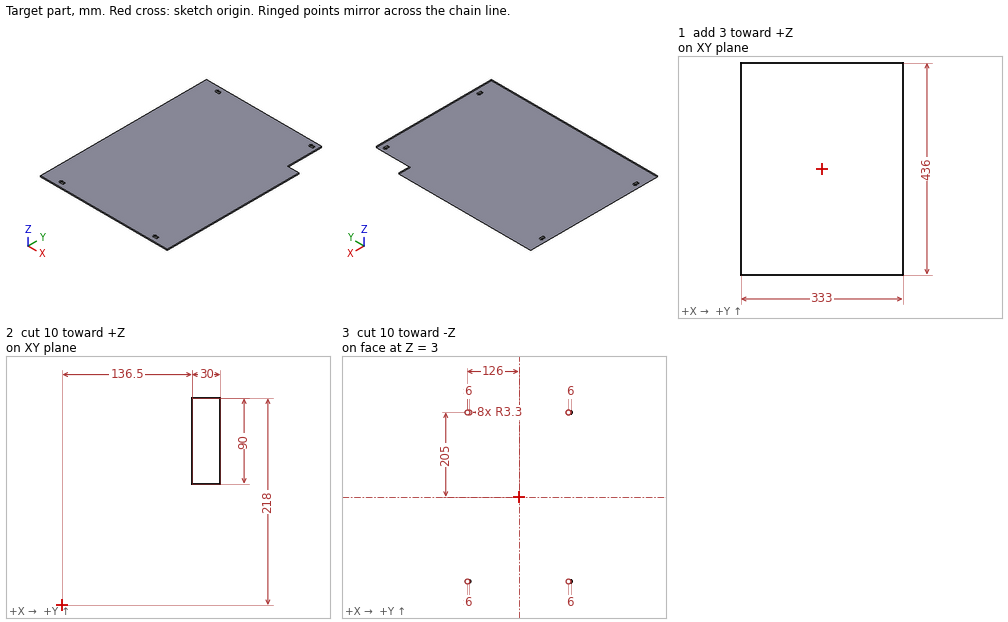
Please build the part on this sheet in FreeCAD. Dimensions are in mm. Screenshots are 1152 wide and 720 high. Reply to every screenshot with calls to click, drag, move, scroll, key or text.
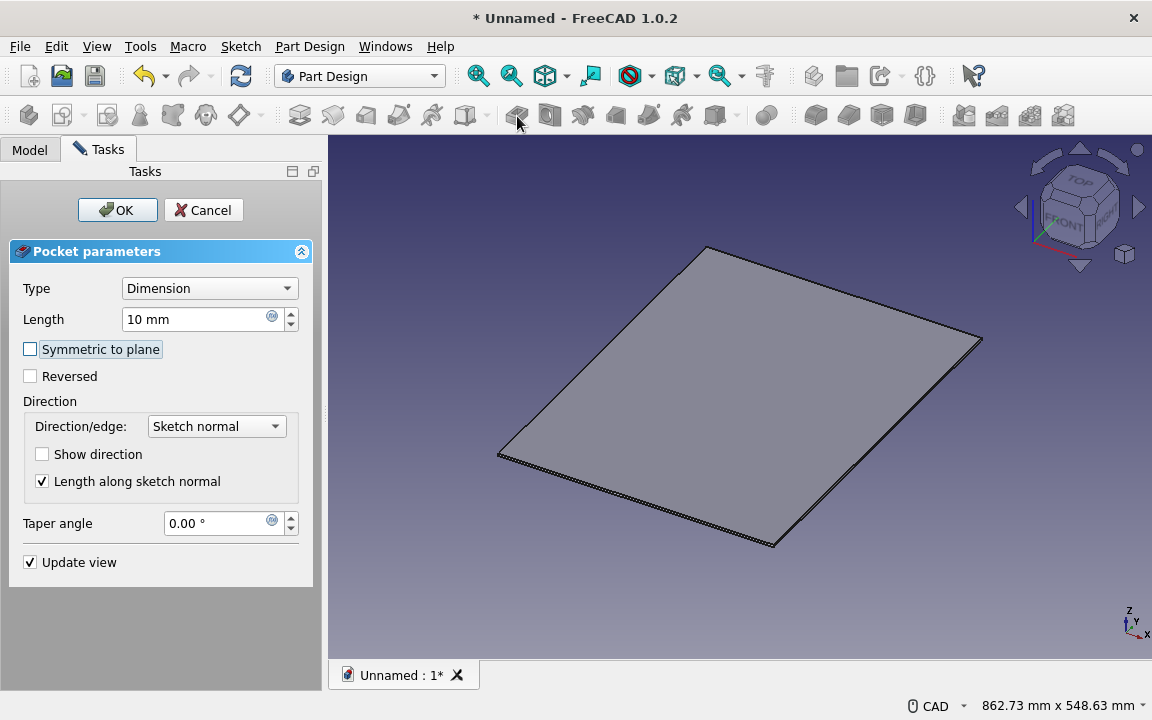
click(31, 376)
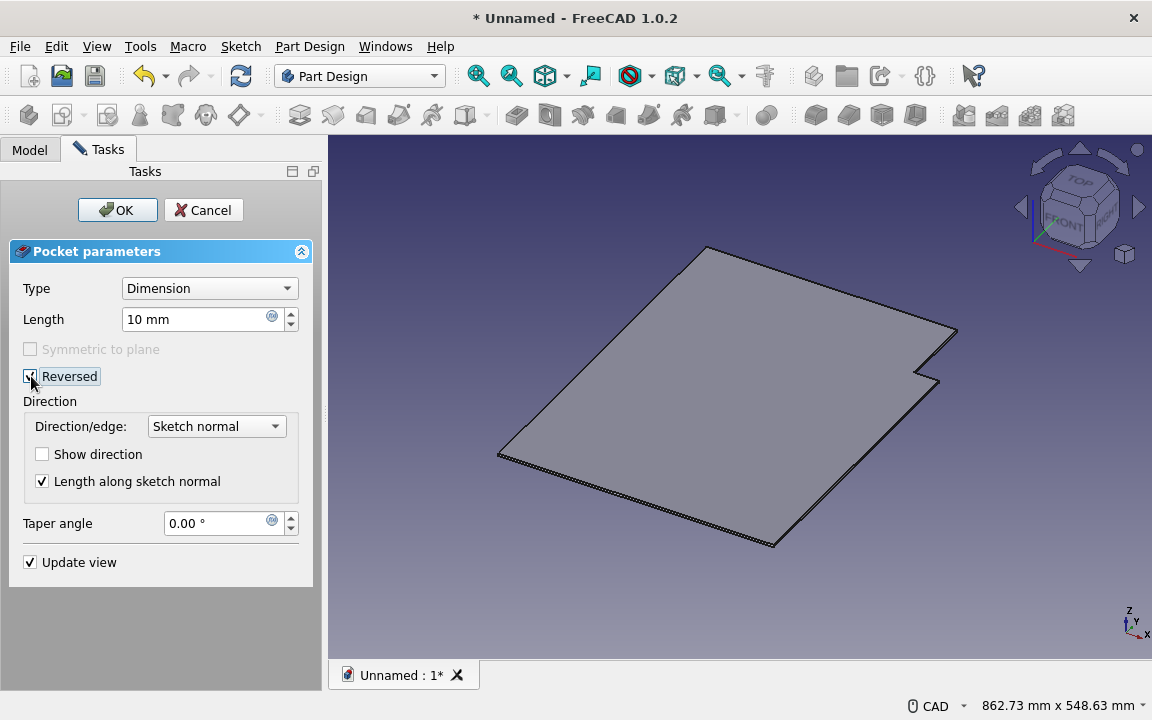
click(118, 210)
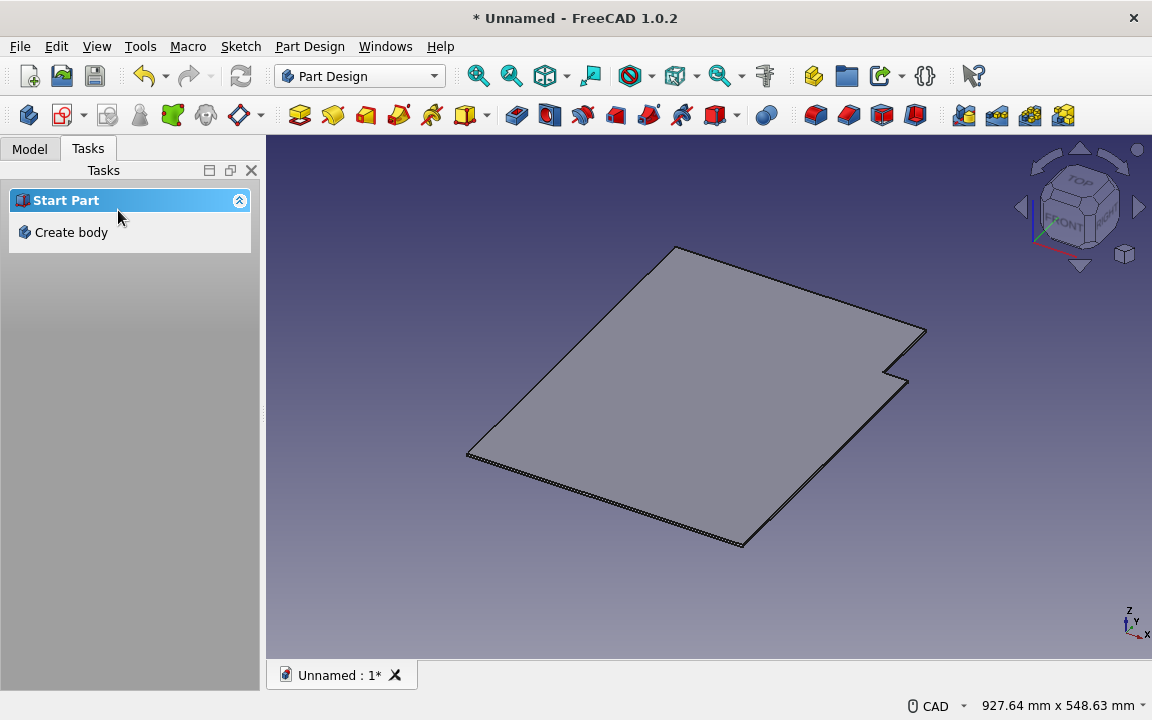
click(709, 395)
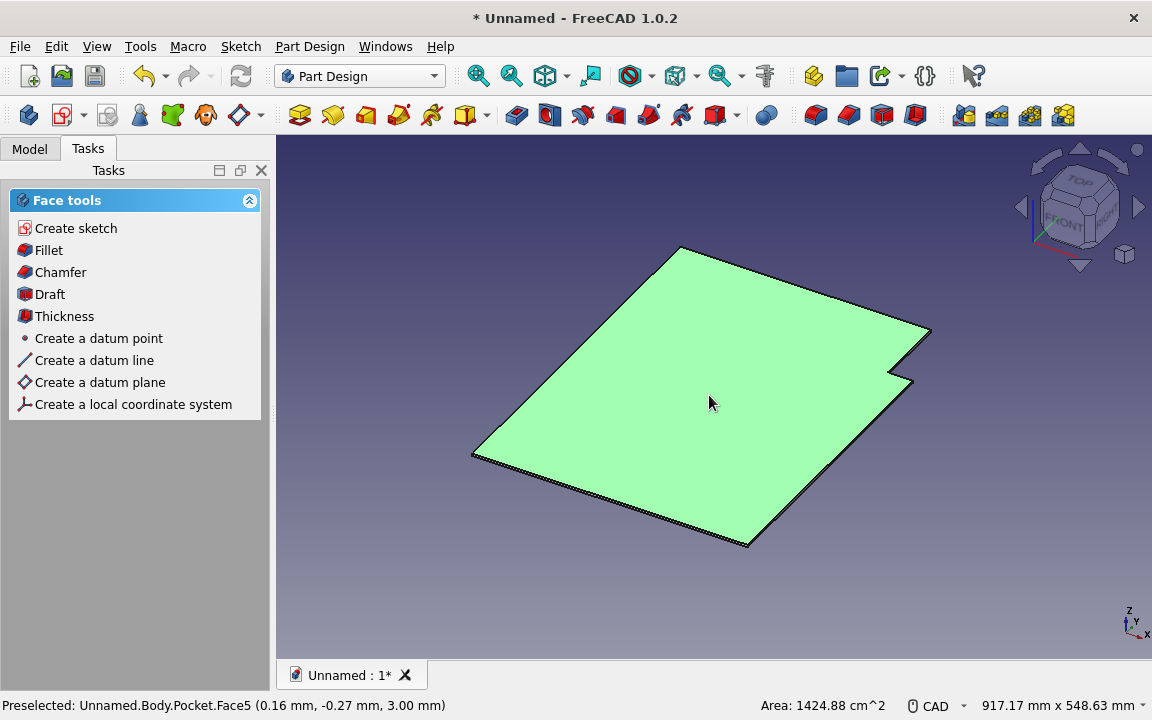
click(62, 116)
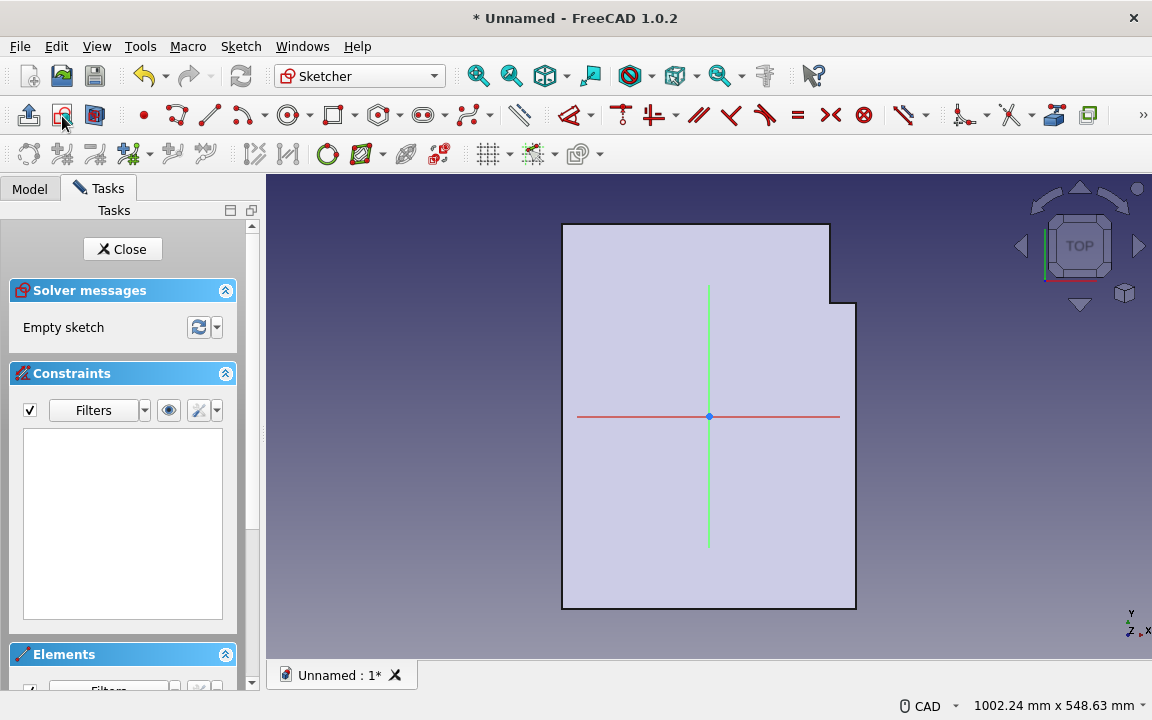
key(g)
key(s)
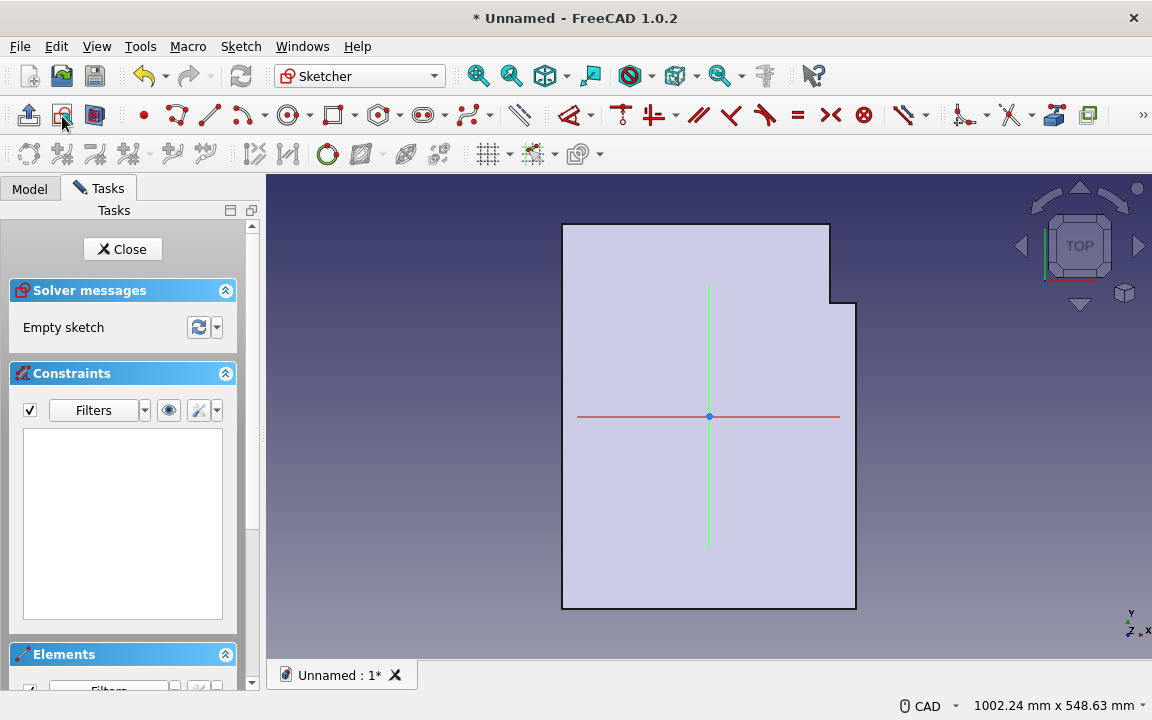
scroll(598, 235, up, 11)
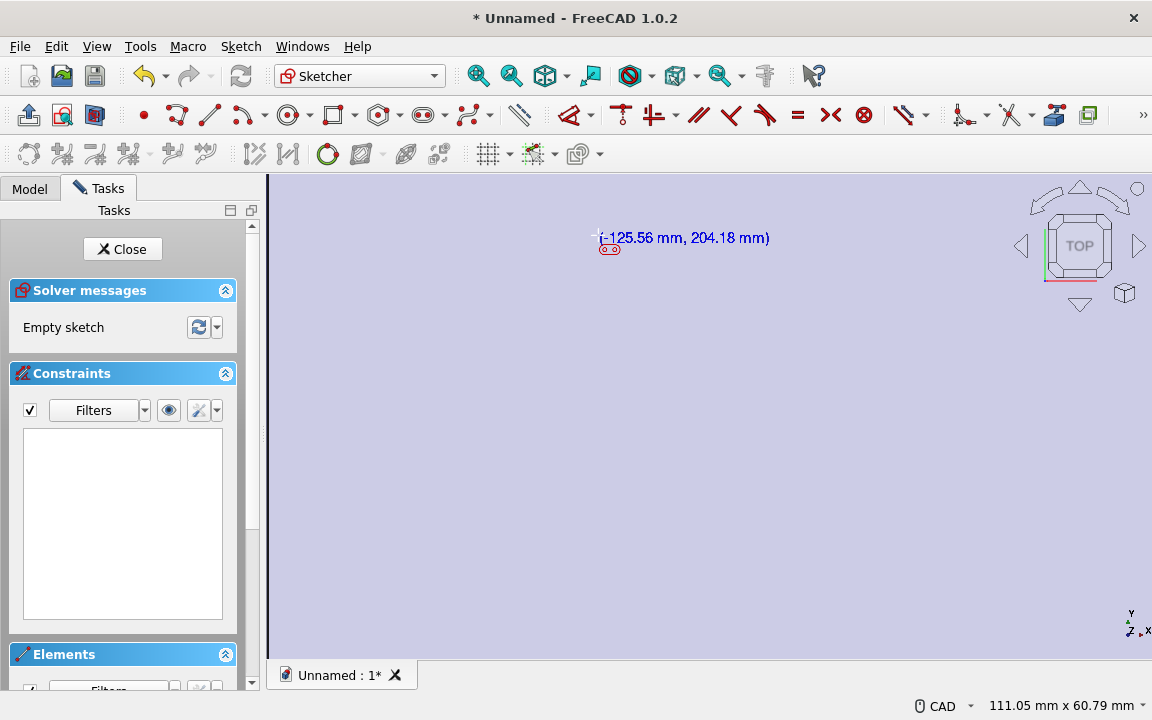
scroll(545, 271, down, 12)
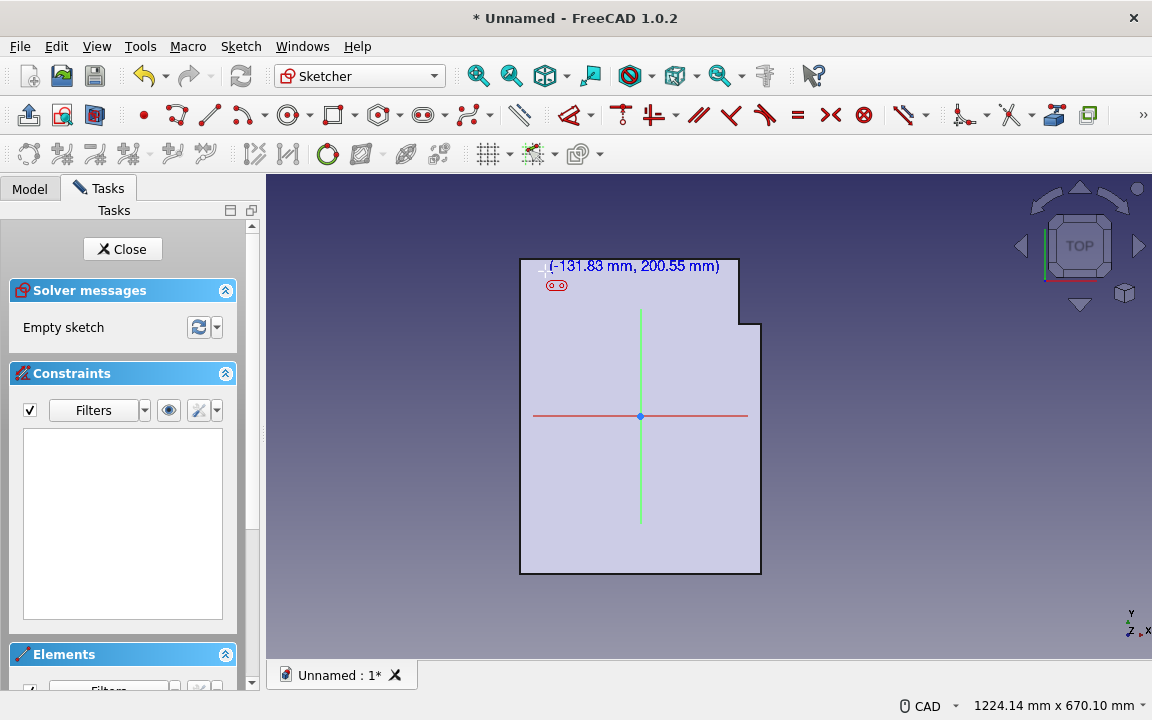
click(550, 268)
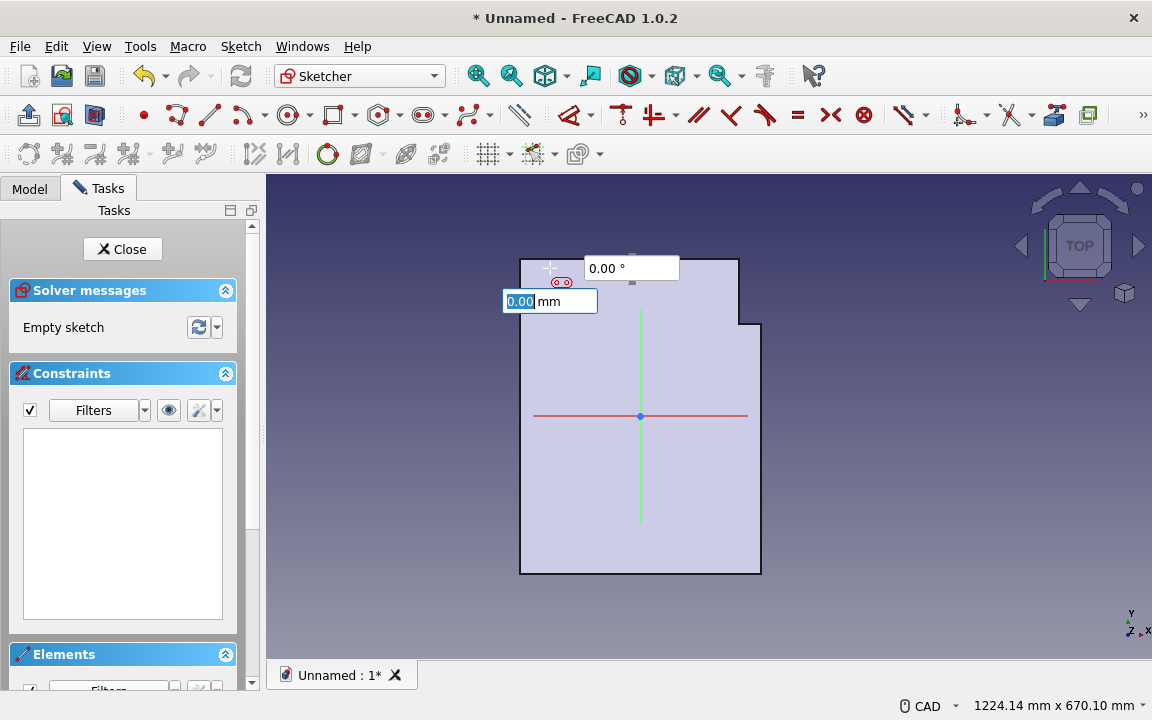
scroll(554, 268, up, 7)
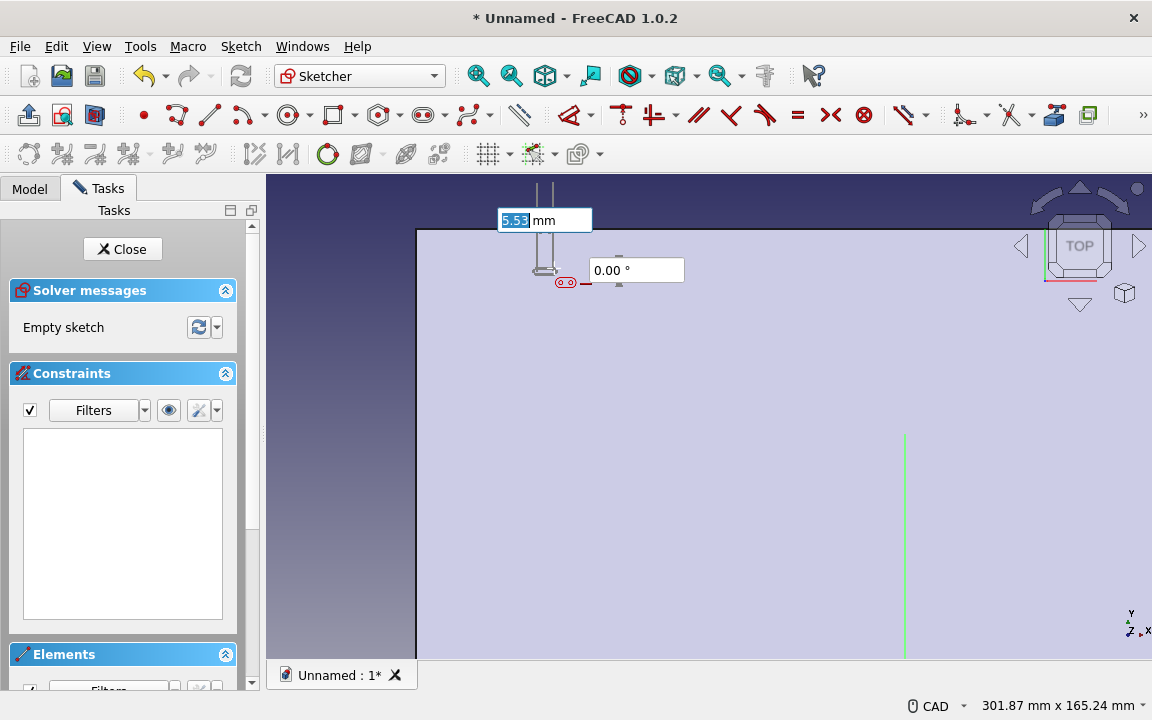
click(552, 267)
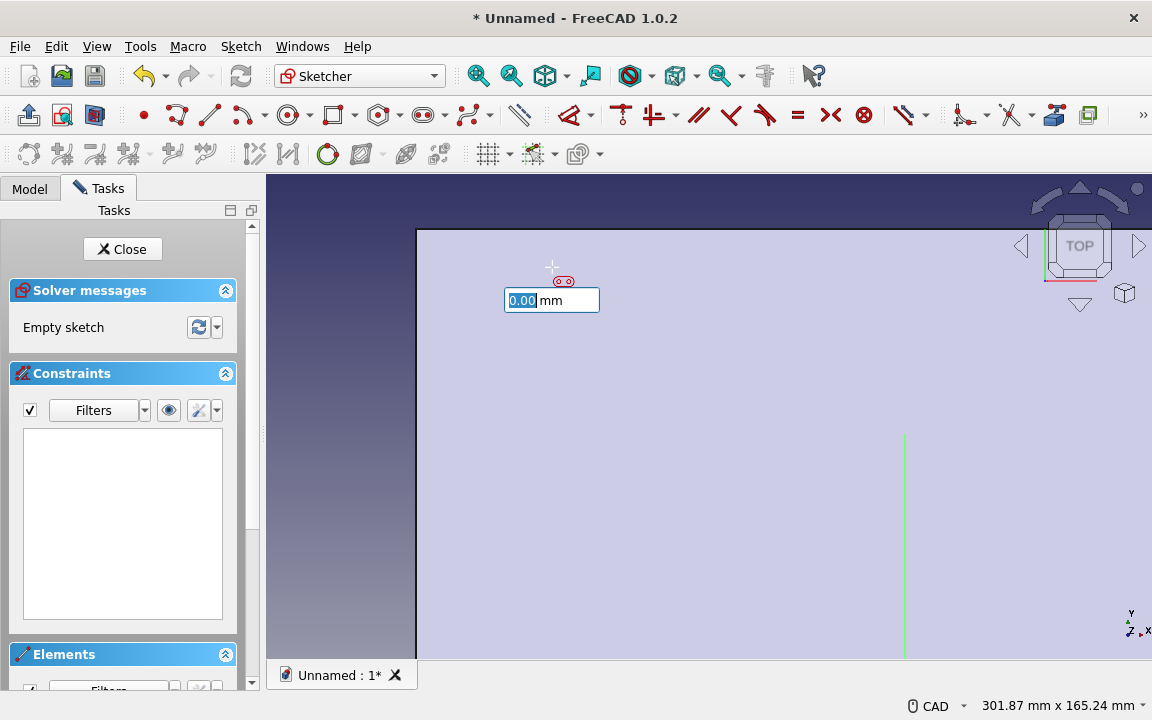
scroll(544, 277, up, 3)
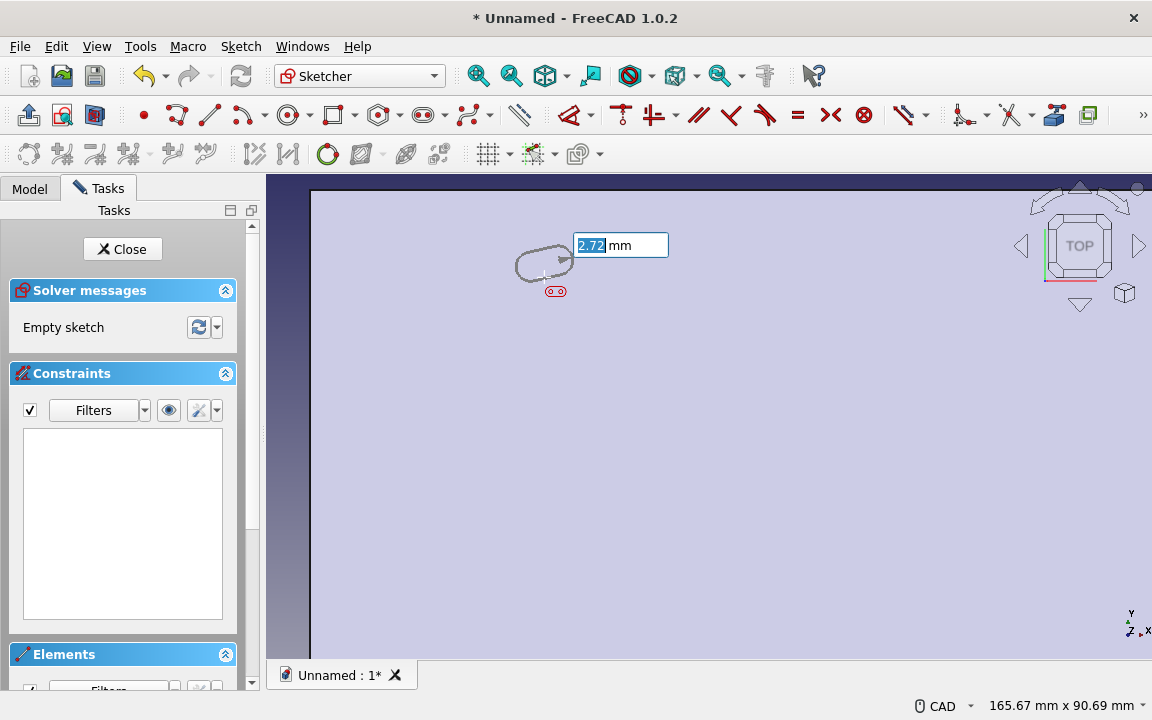
click(543, 277)